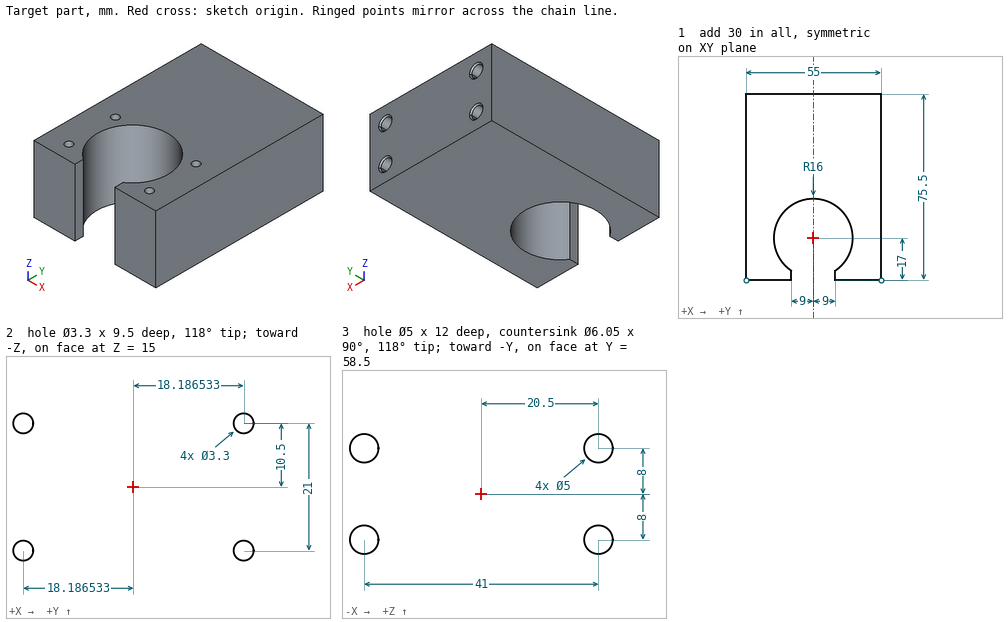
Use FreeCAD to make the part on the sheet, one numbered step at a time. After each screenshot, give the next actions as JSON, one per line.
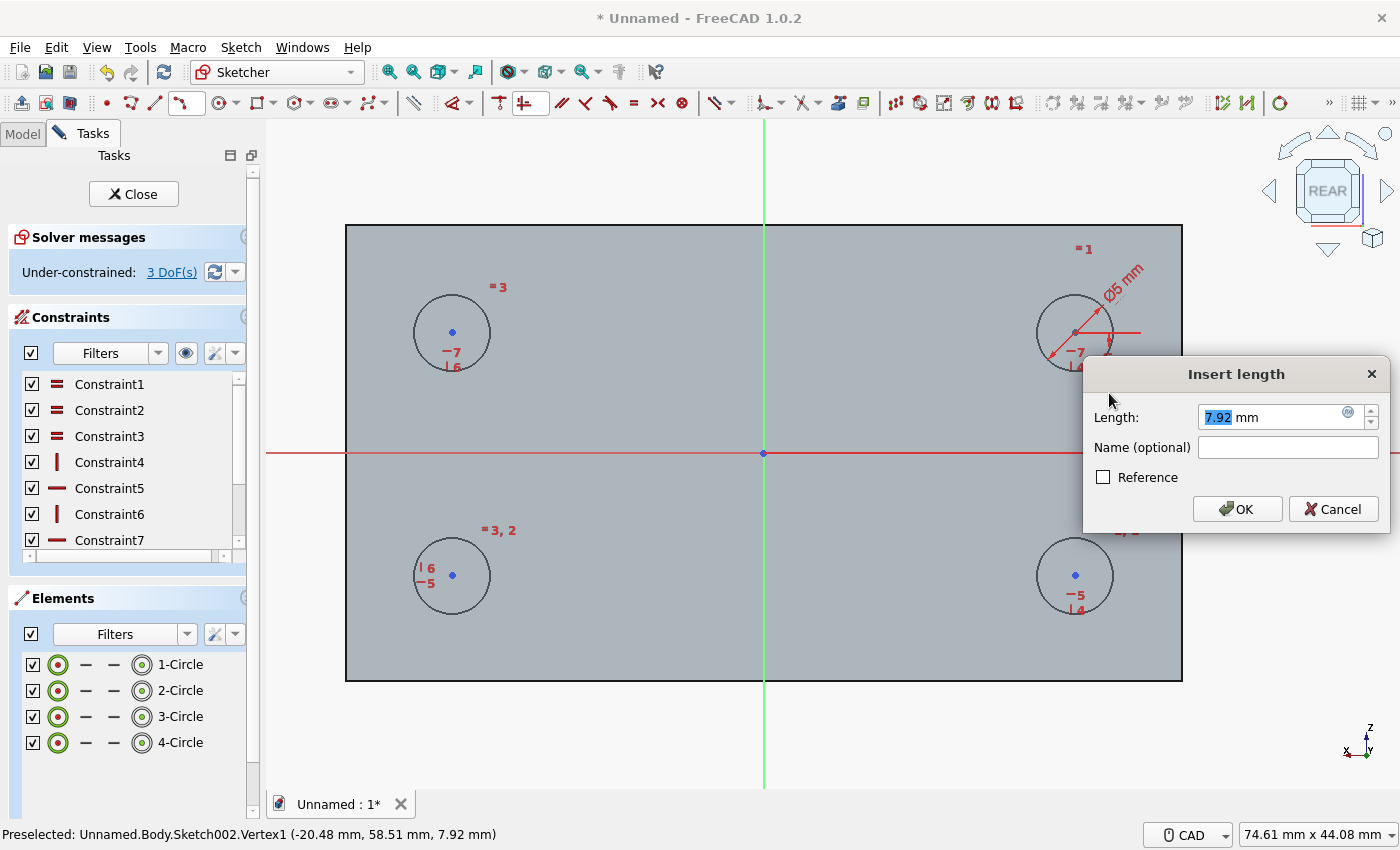
{"action": "type", "text": "8"}
{"action": "key", "text": "Return"}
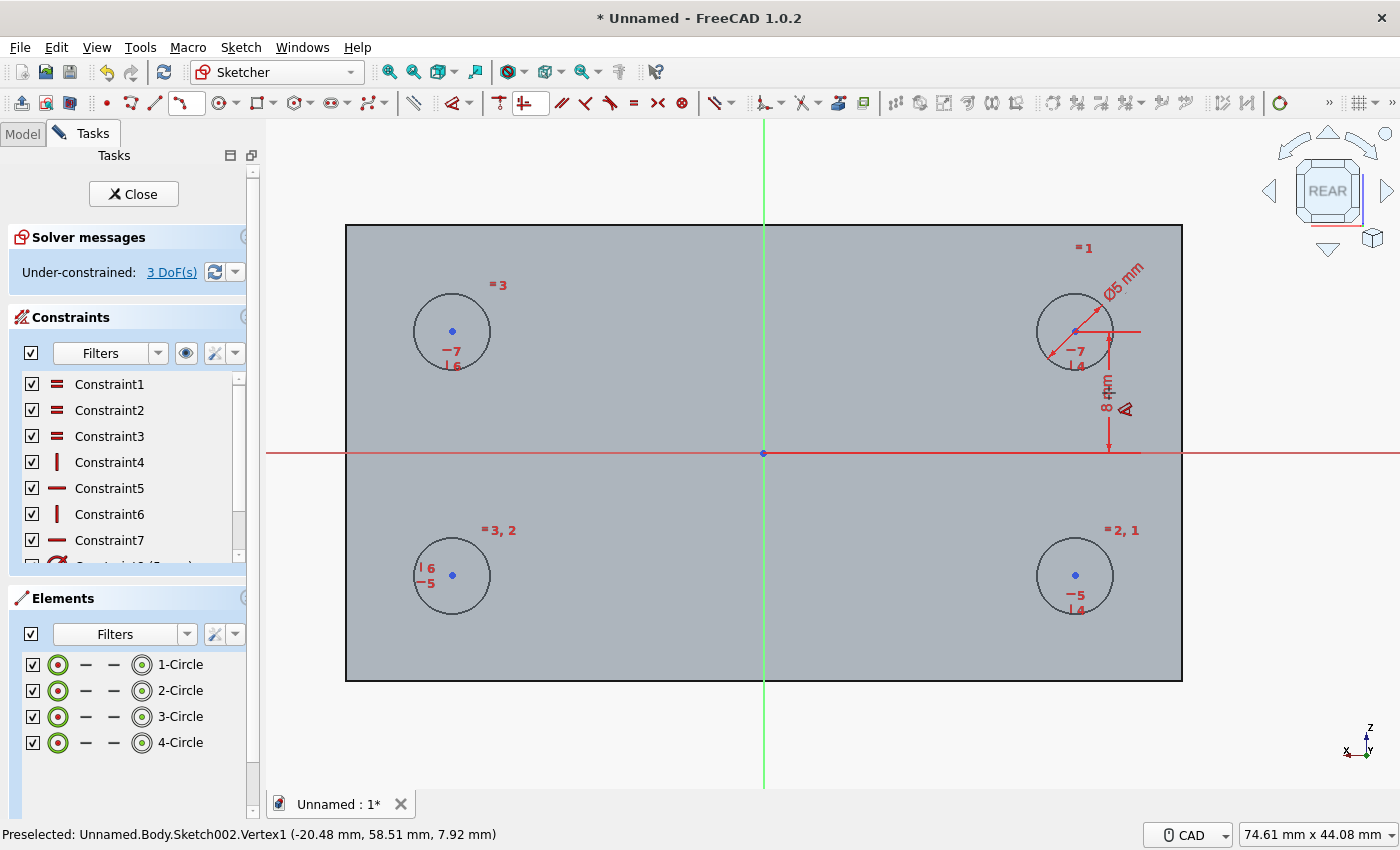
{"action": "left_click", "coordinate": [1075, 576]}
{"action": "left_click", "coordinate": [1109, 515]}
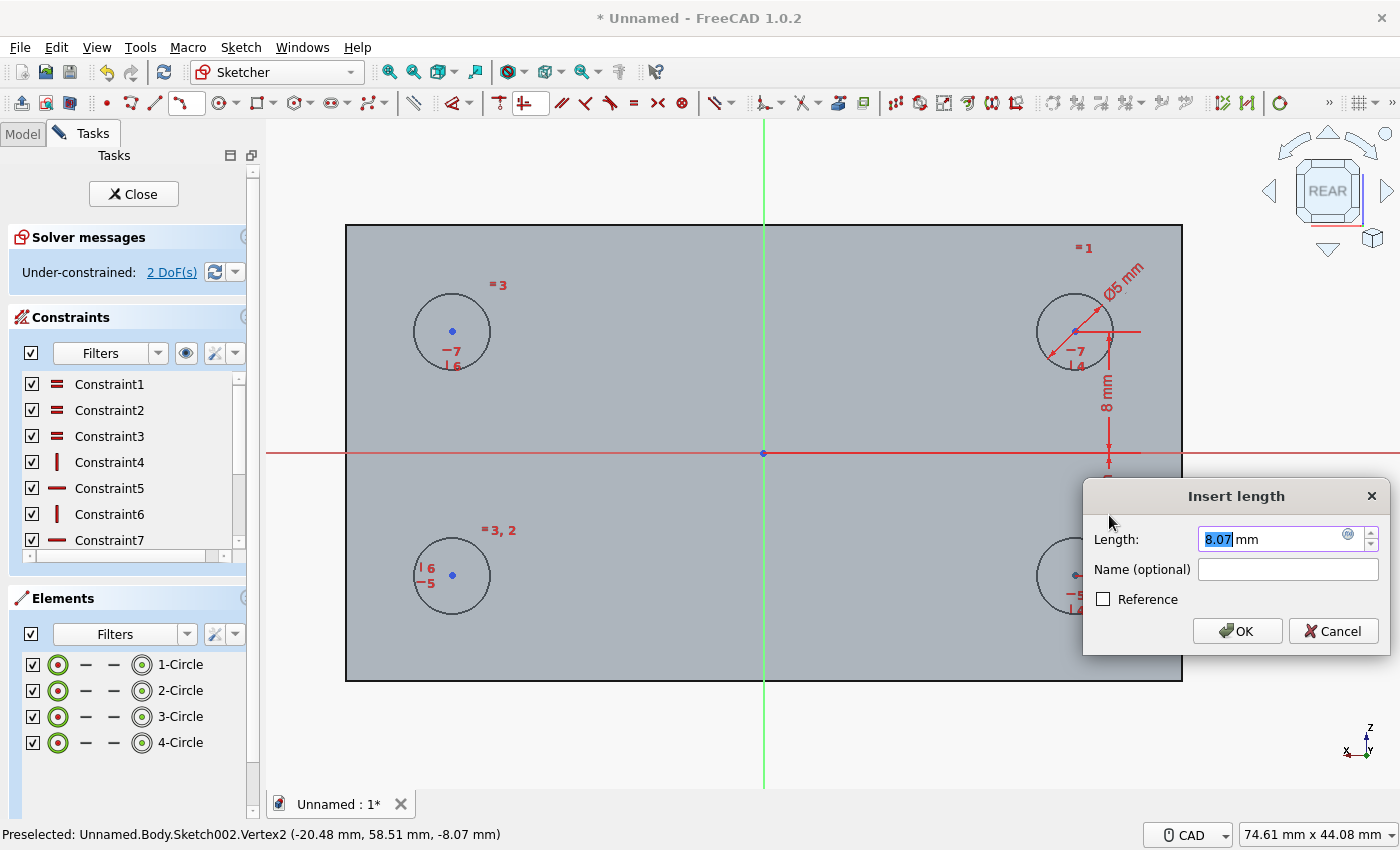
{"action": "type", "text": "8"}
{"action": "key", "text": "Return"}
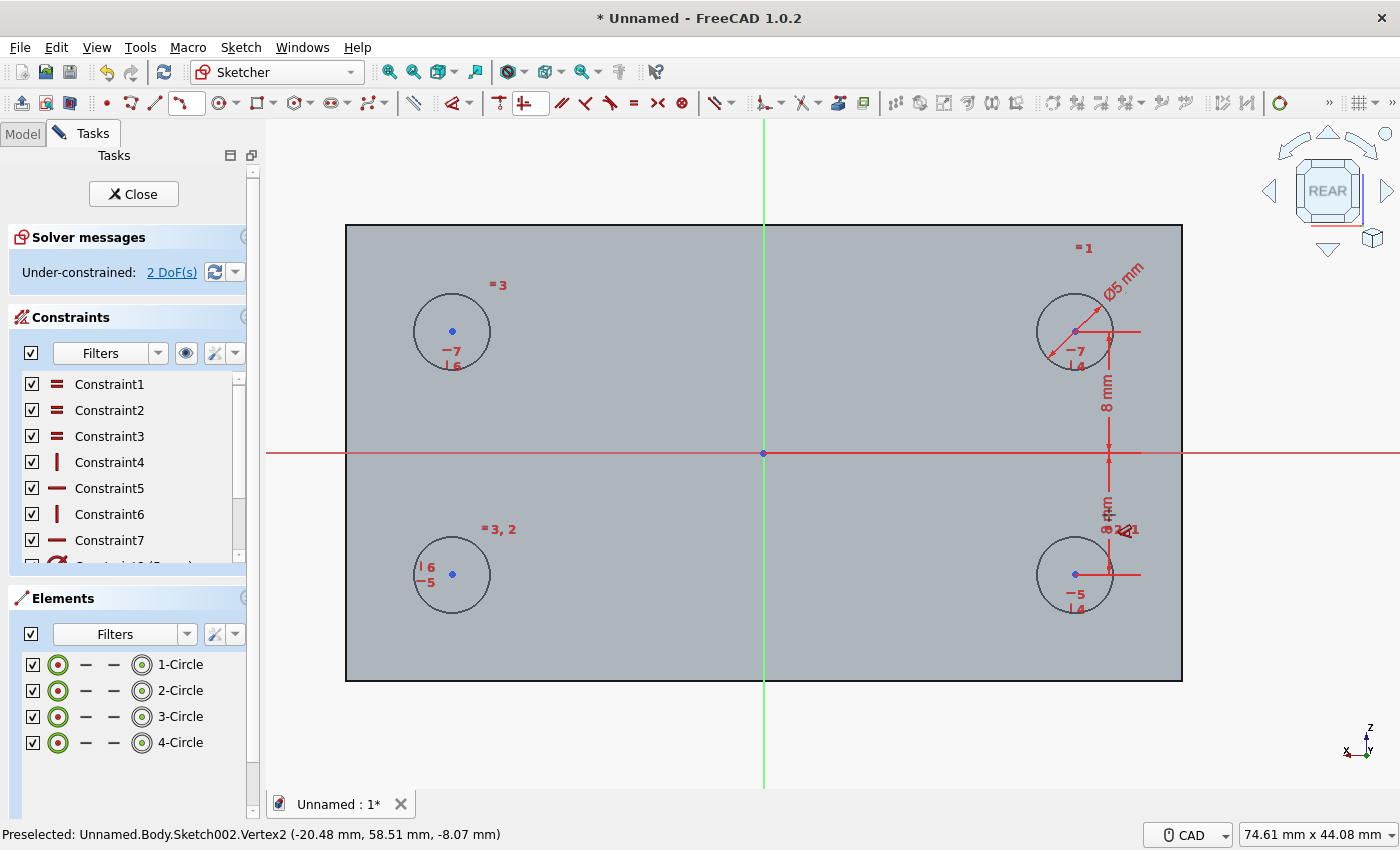
{"action": "left_click", "coordinate": [1075, 575]}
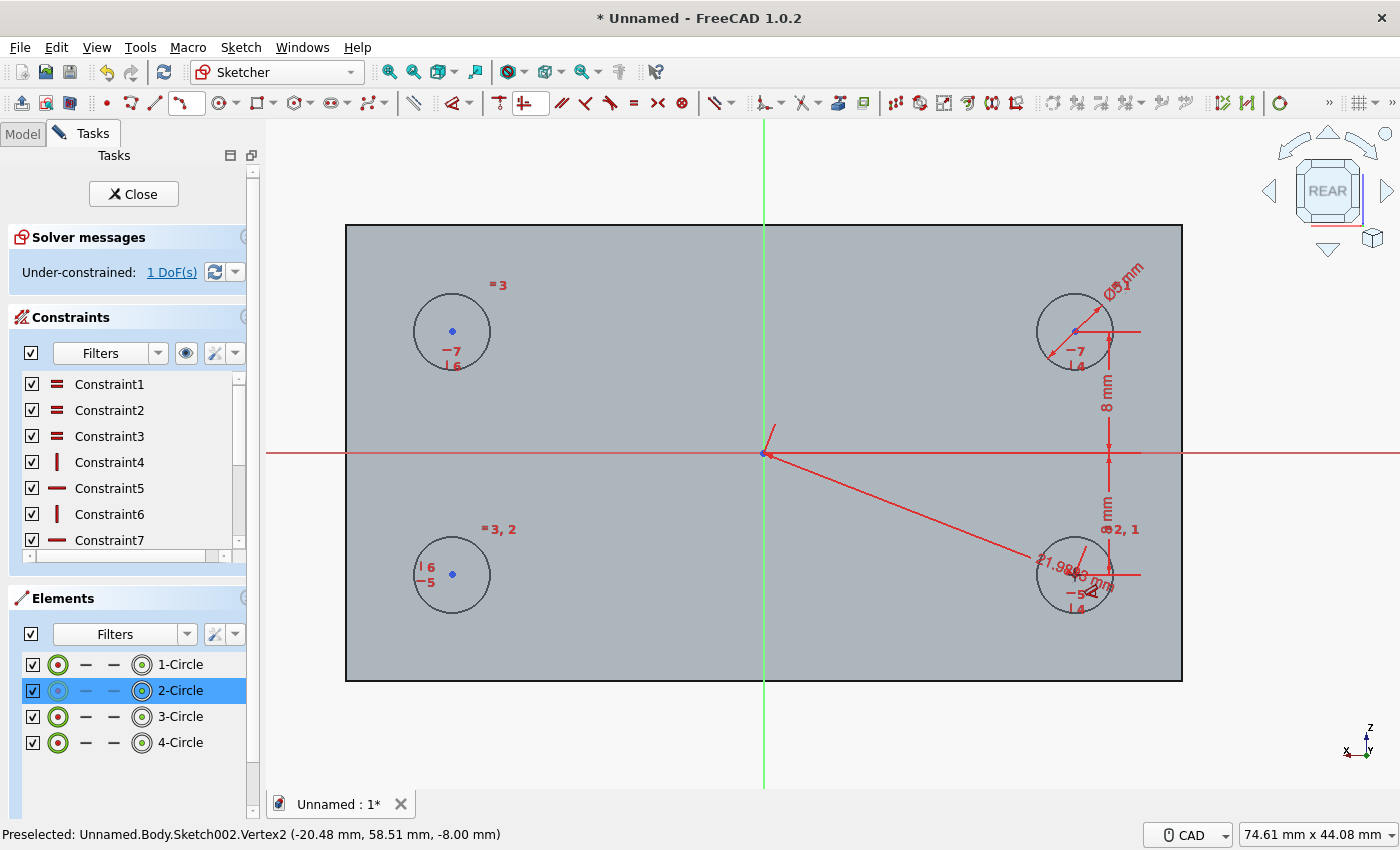
{"action": "left_click", "coordinate": [452, 575]}
{"action": "left_click", "coordinate": [620, 609]}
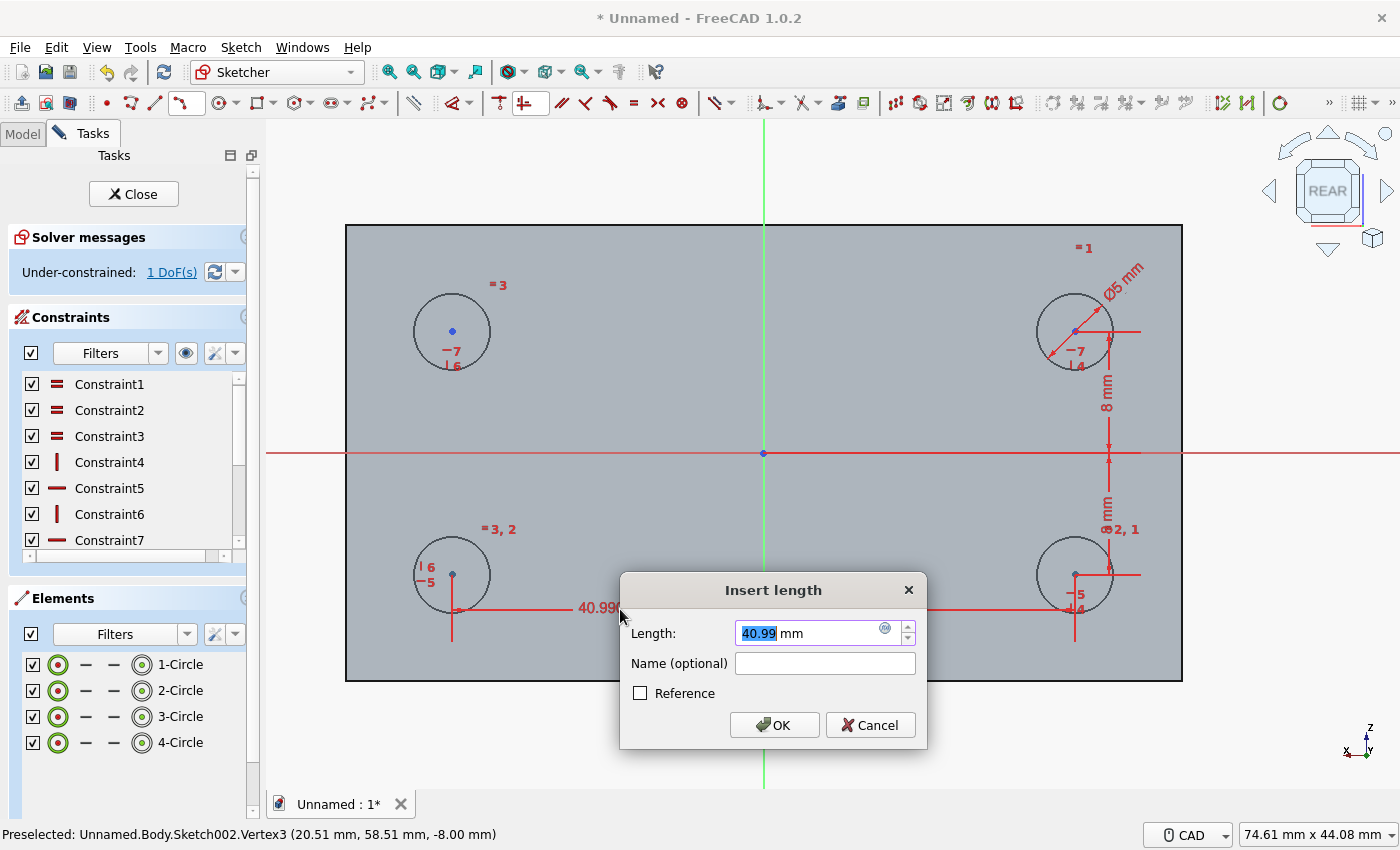
{"action": "type", "text": "41"}
{"action": "key", "text": "Return"}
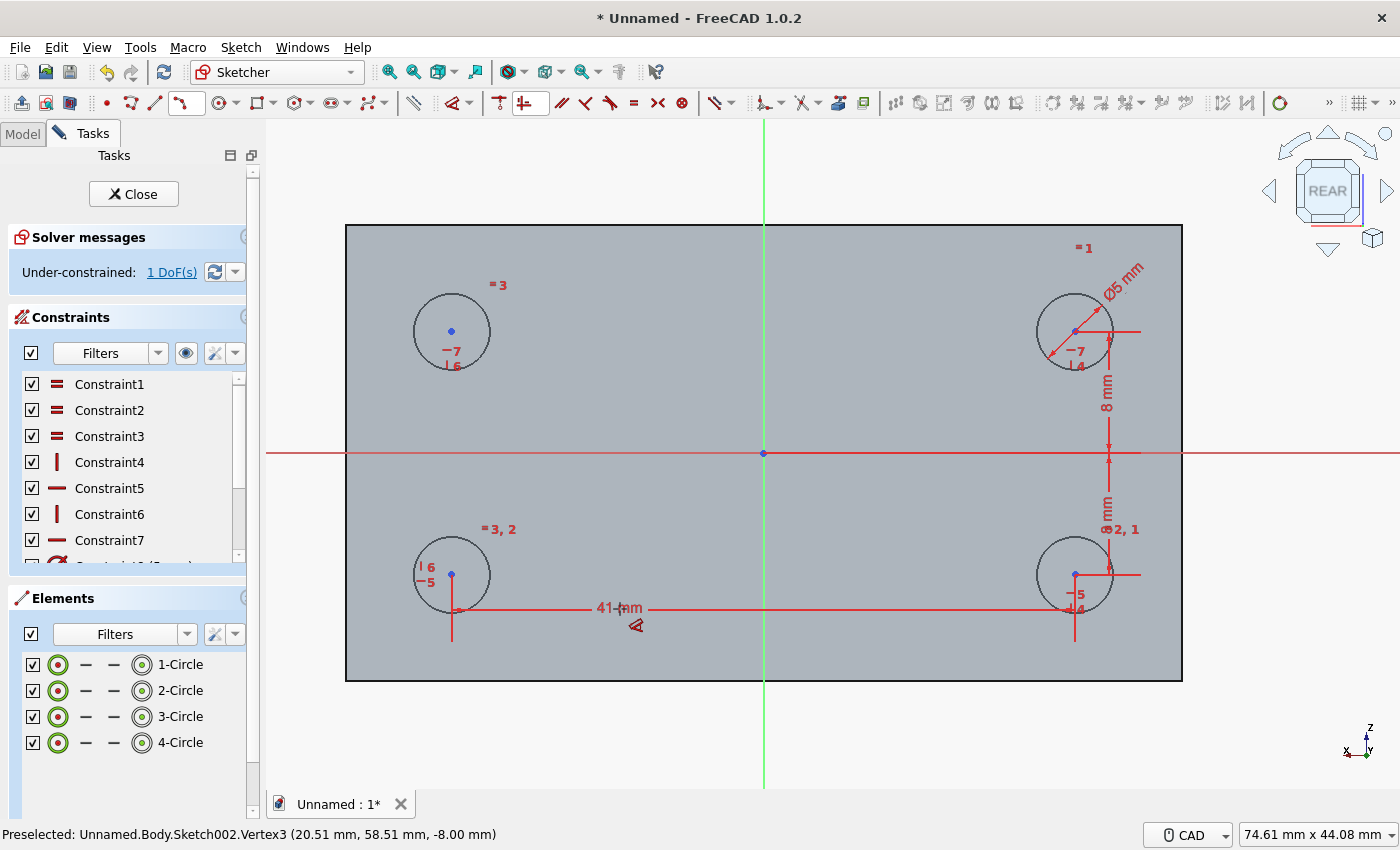
{"action": "left_click", "coordinate": [1075, 332]}
{"action": "left_click", "coordinate": [919, 298]}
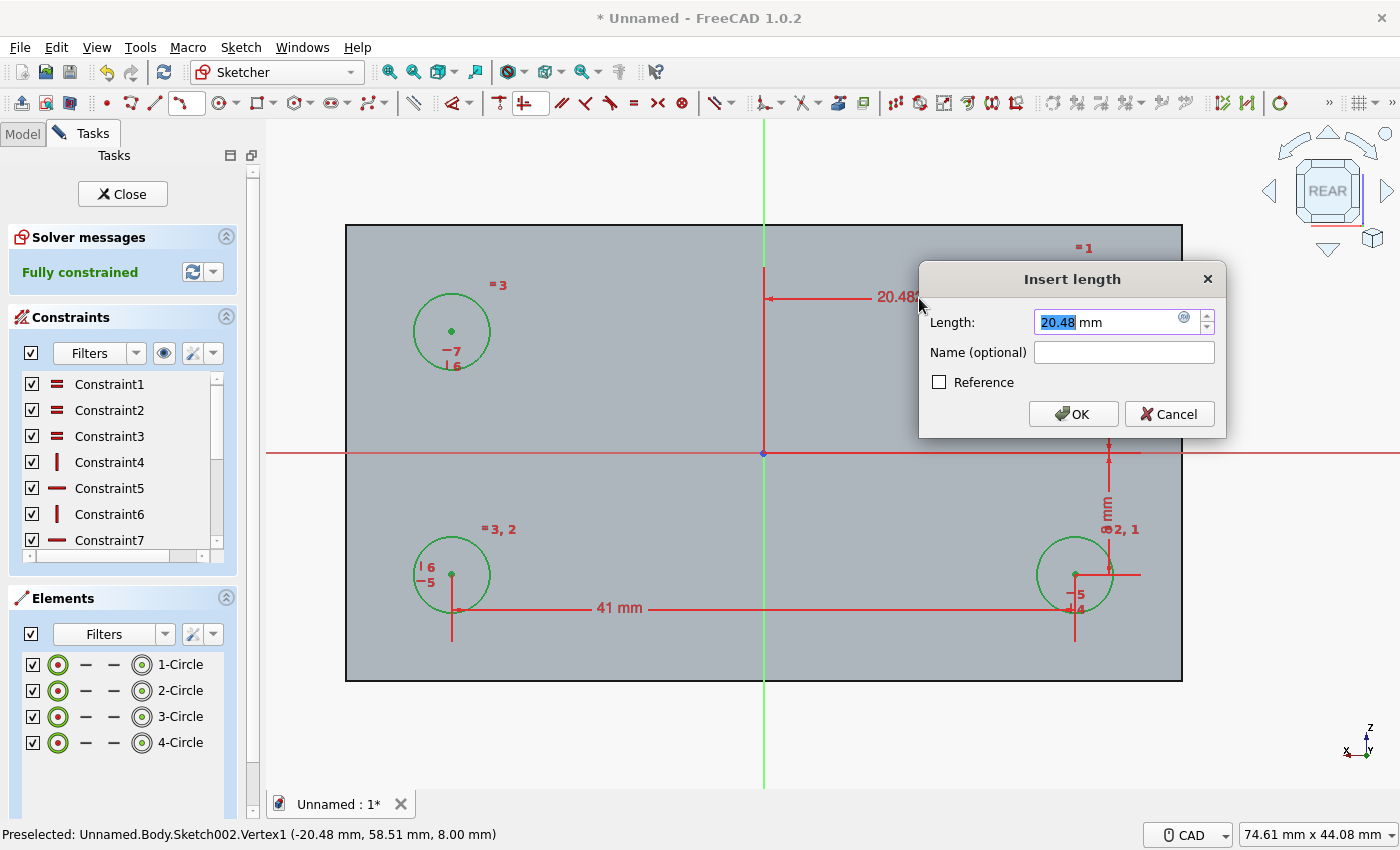
{"action": "type", "text": "20.5"}
{"action": "key", "text": "Return"}
{"action": "key", "text": "Escape"}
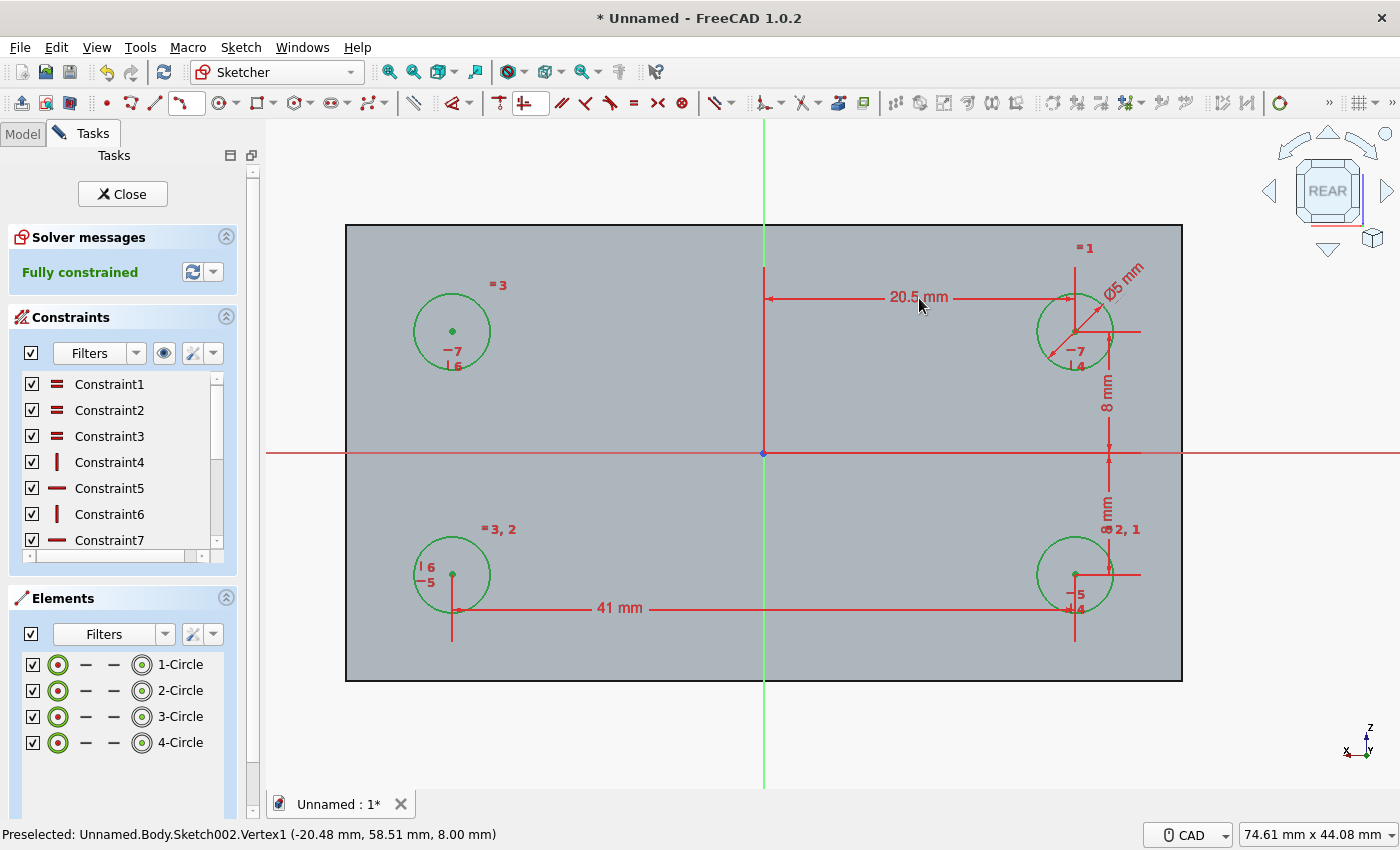
{"action": "left_click", "coordinate": [123, 194]}